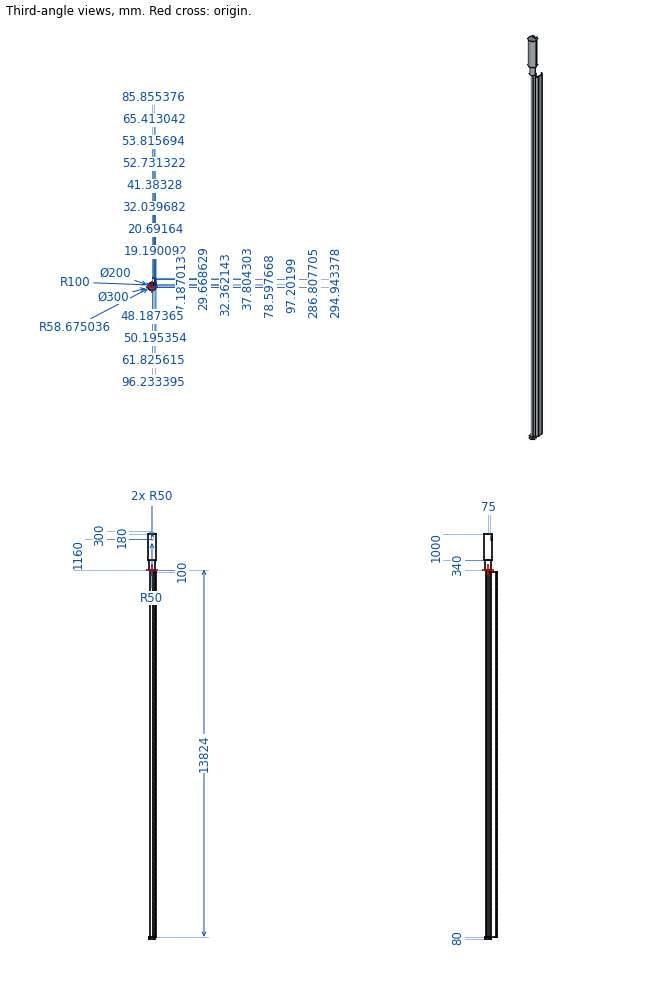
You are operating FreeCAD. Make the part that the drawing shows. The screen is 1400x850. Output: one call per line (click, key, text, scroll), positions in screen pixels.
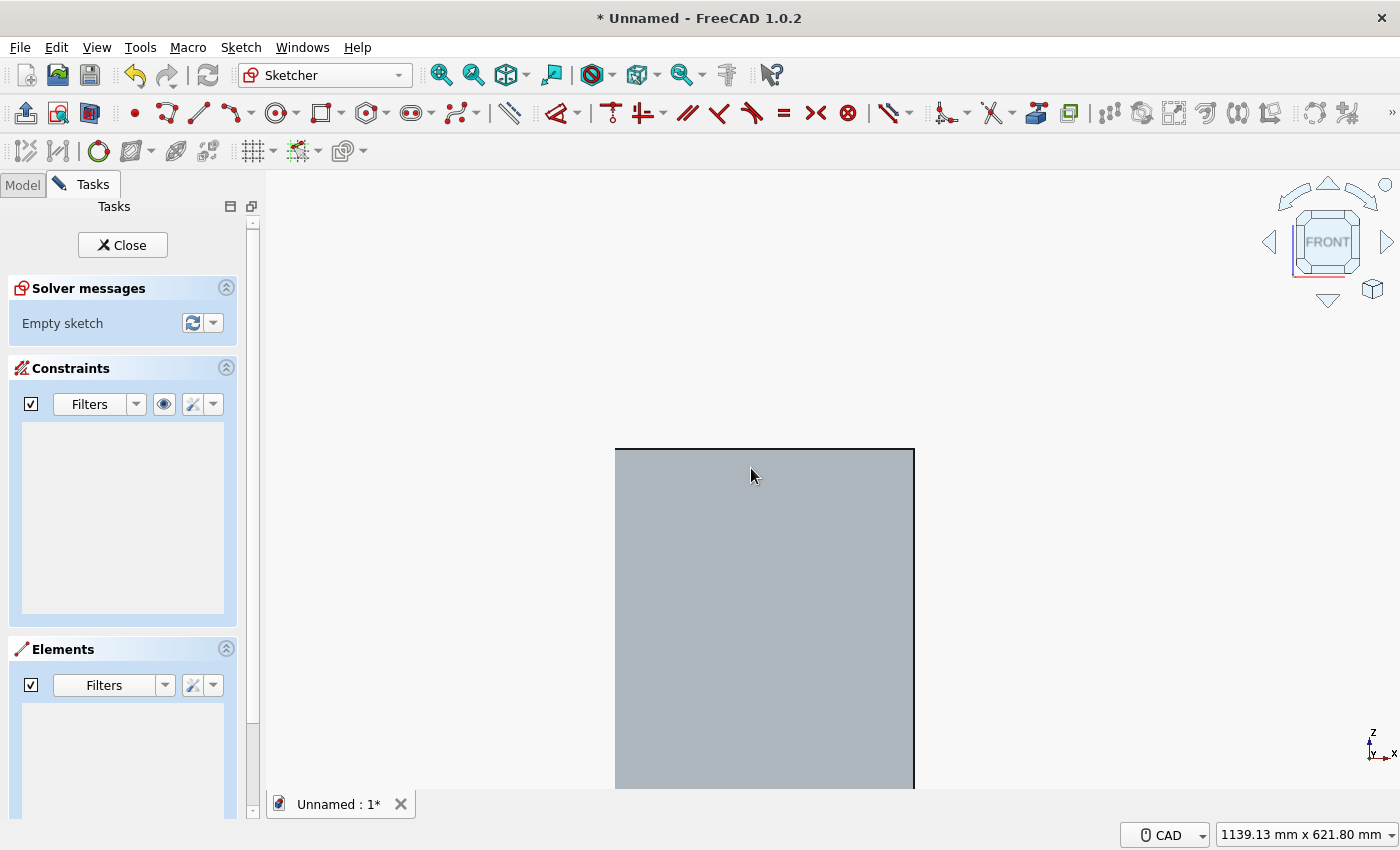
click(764, 628)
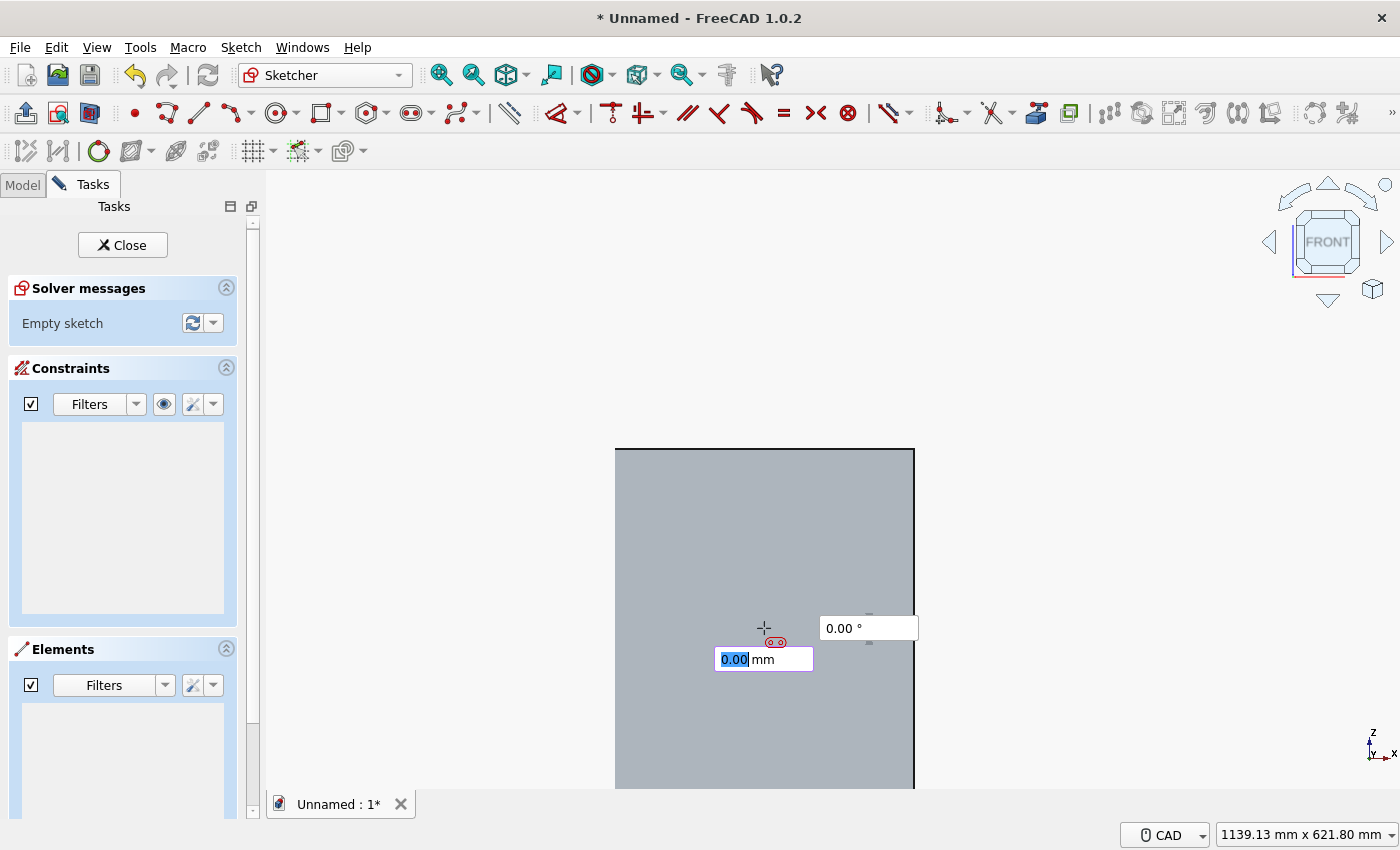
click(773, 329)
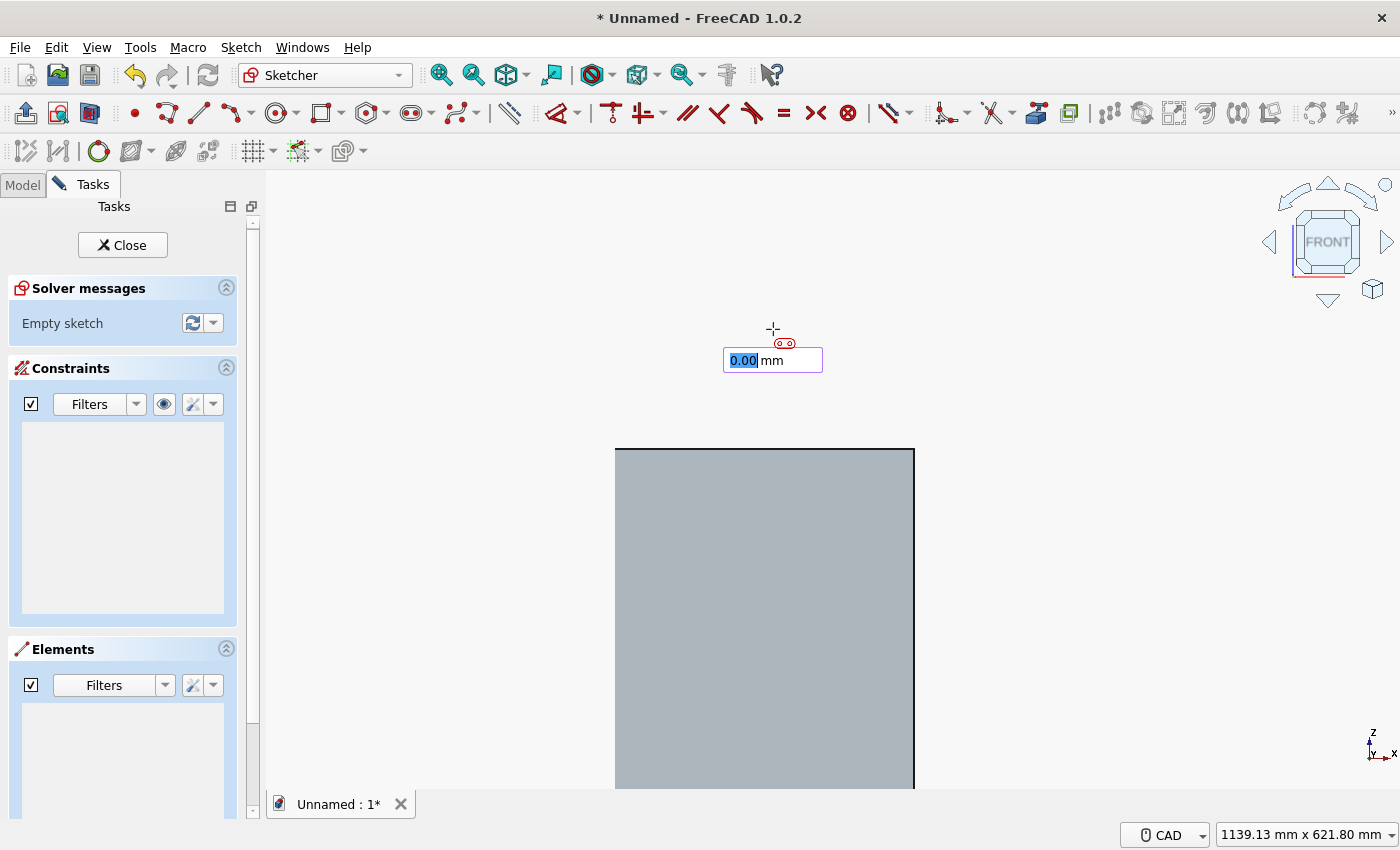
click(814, 479)
key(Escape)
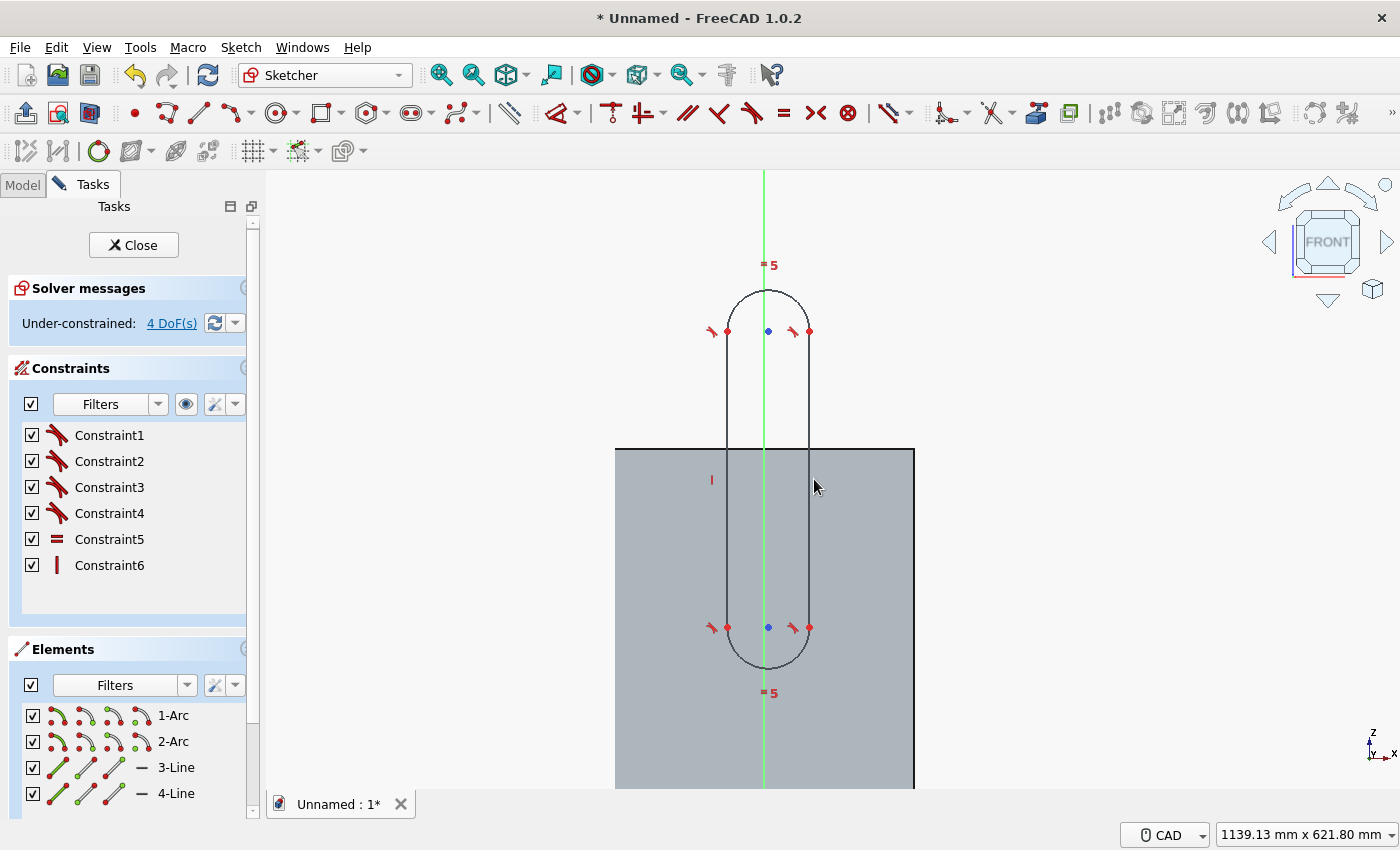
click(768, 628)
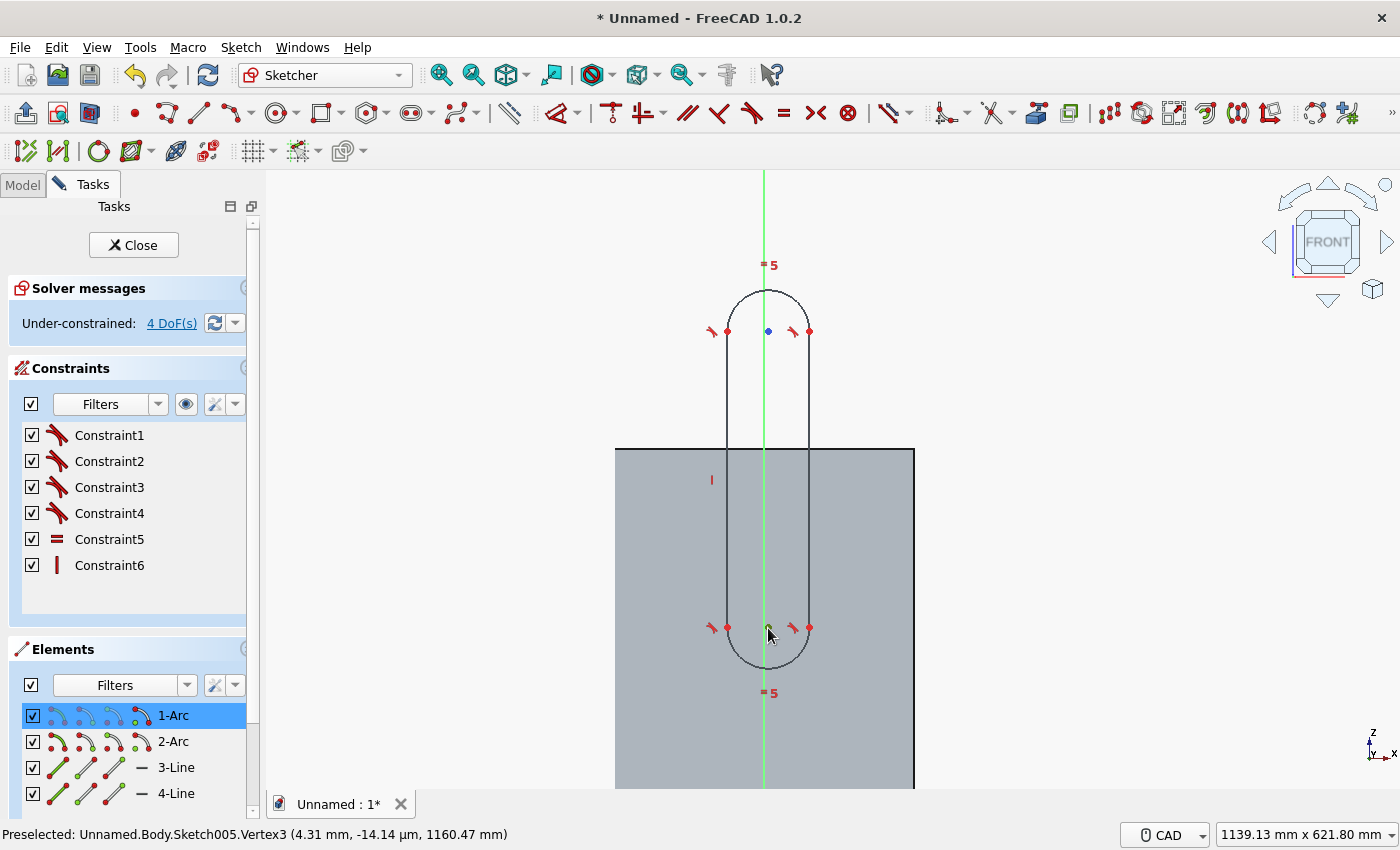
click(764, 721)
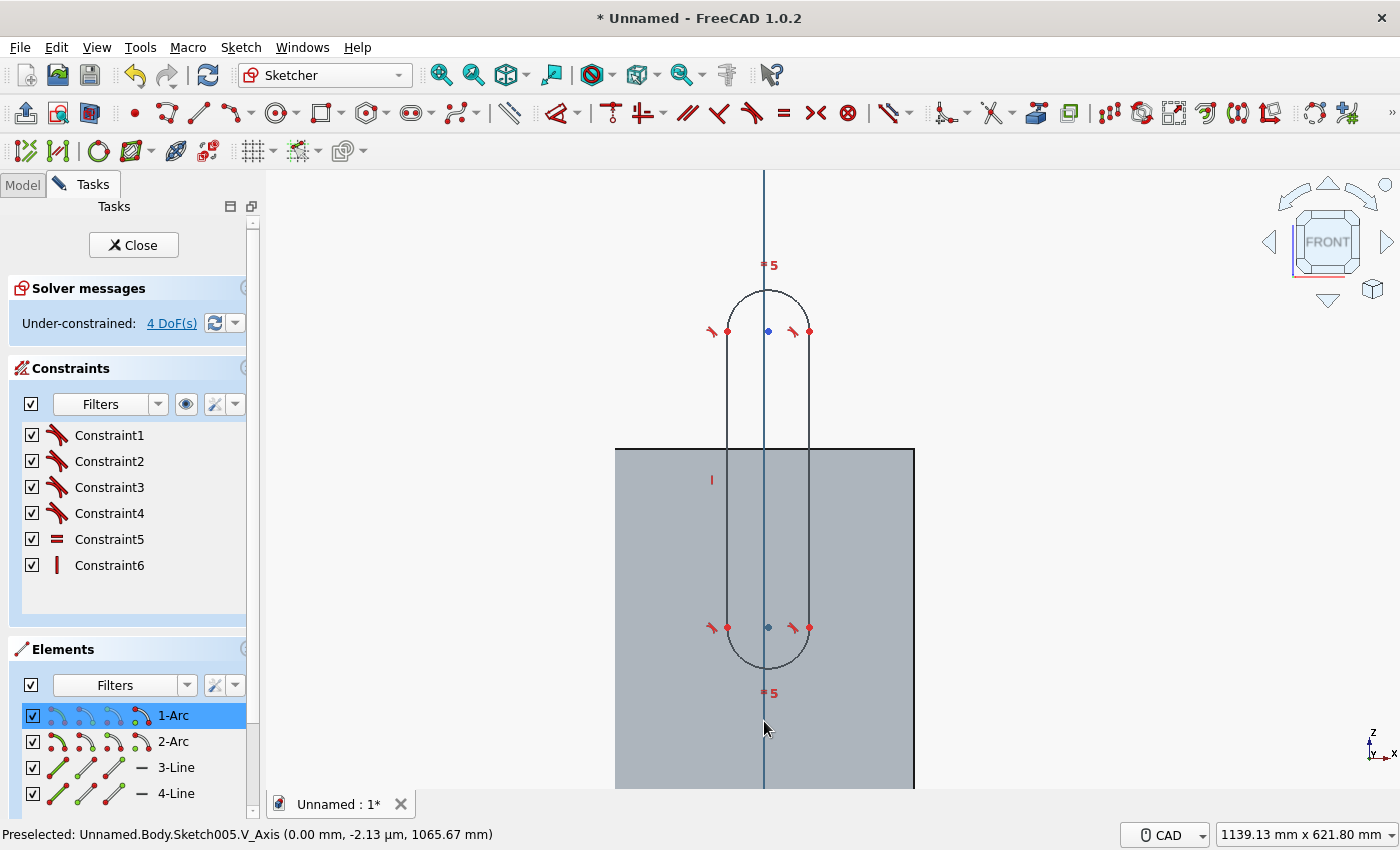
key(c)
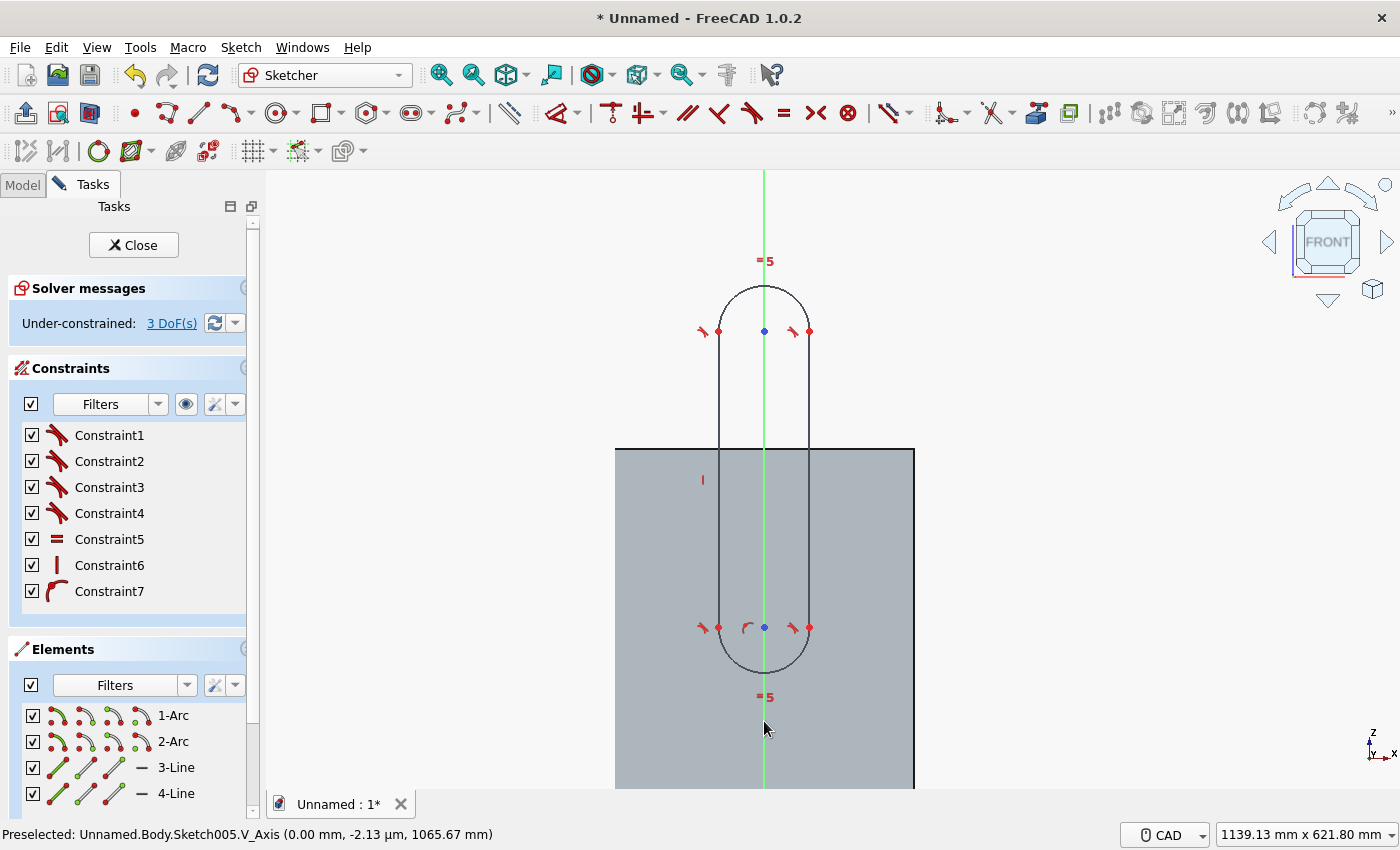
key(d)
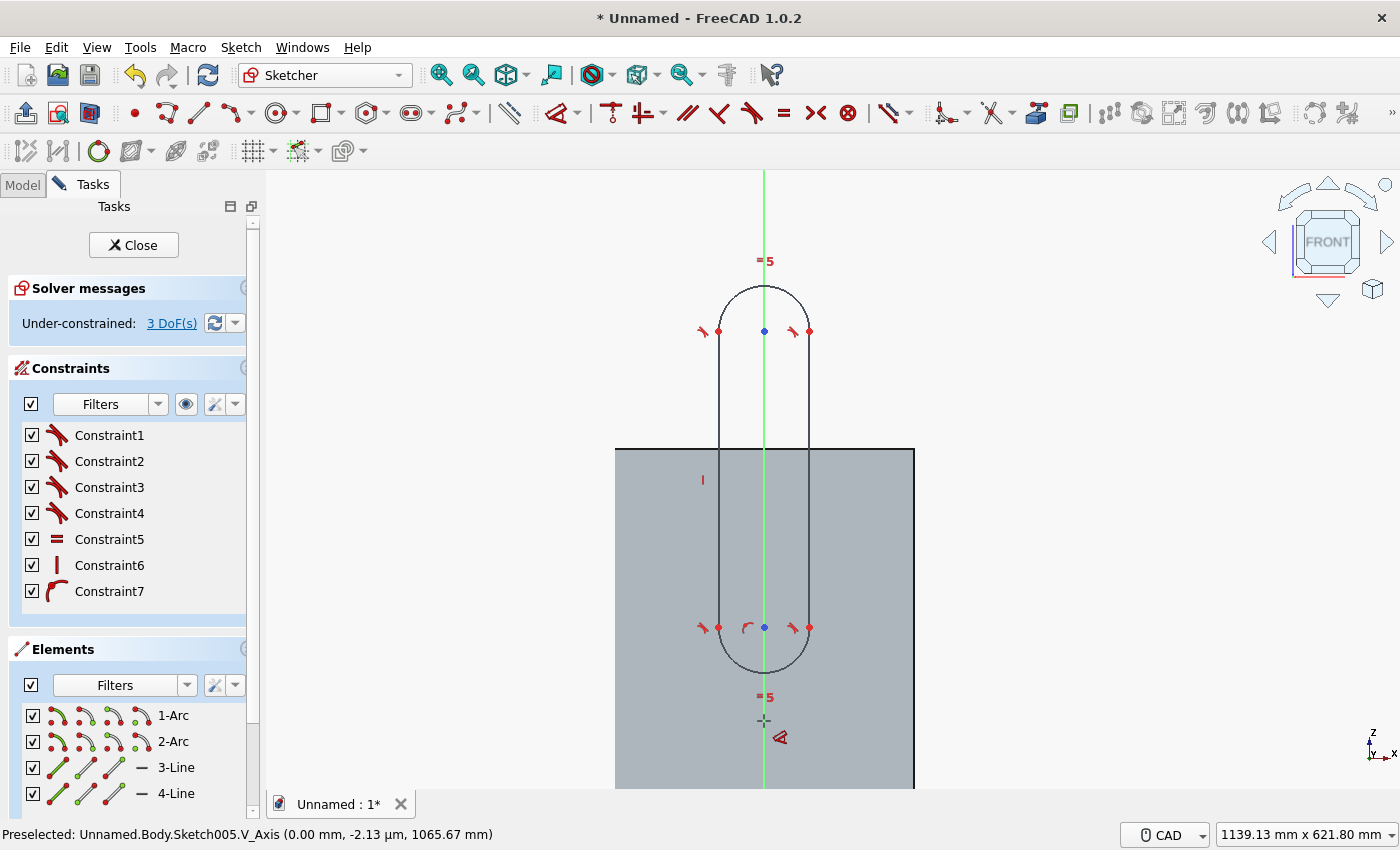
click(738, 664)
click(719, 690)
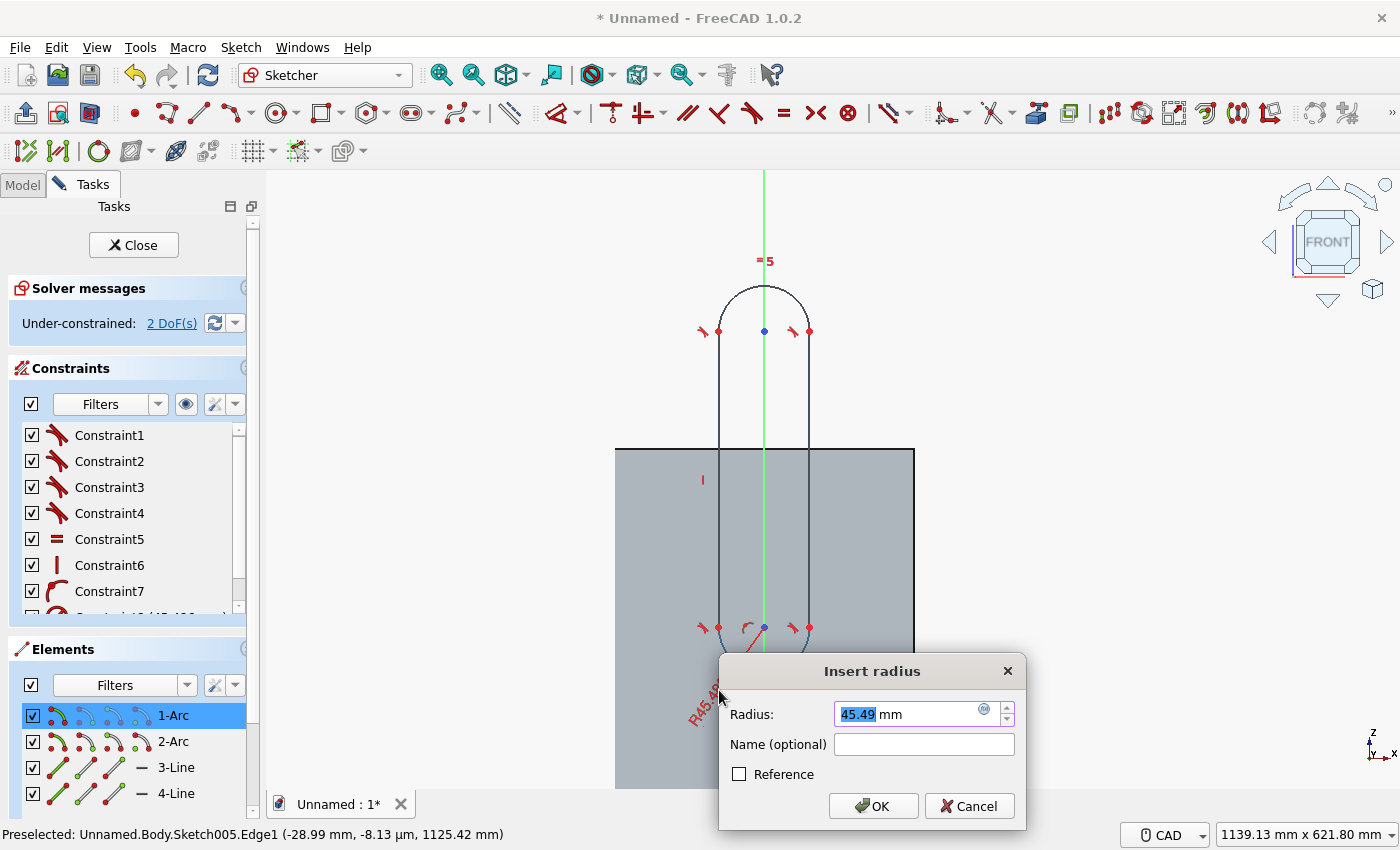
text(50)
key(Return)